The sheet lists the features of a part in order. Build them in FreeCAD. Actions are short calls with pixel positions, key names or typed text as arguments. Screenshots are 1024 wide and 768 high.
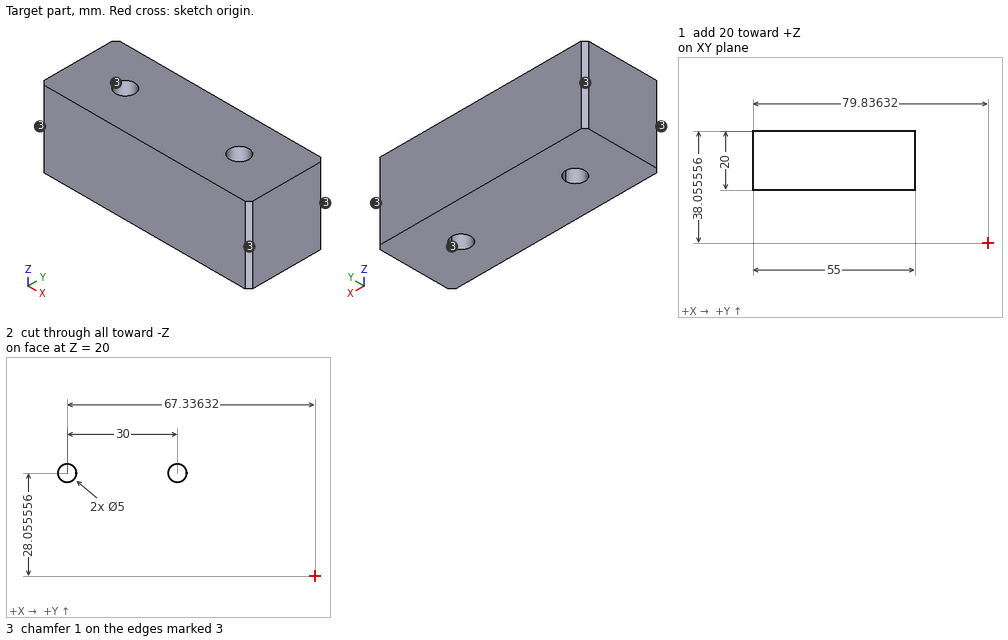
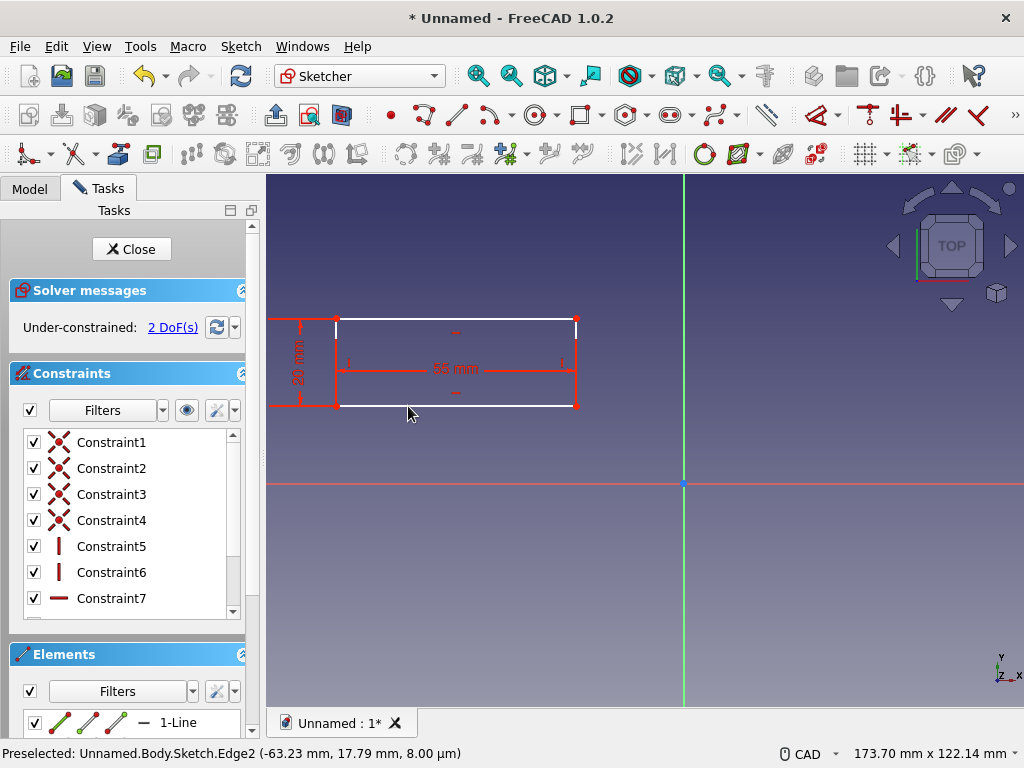
click(336, 319)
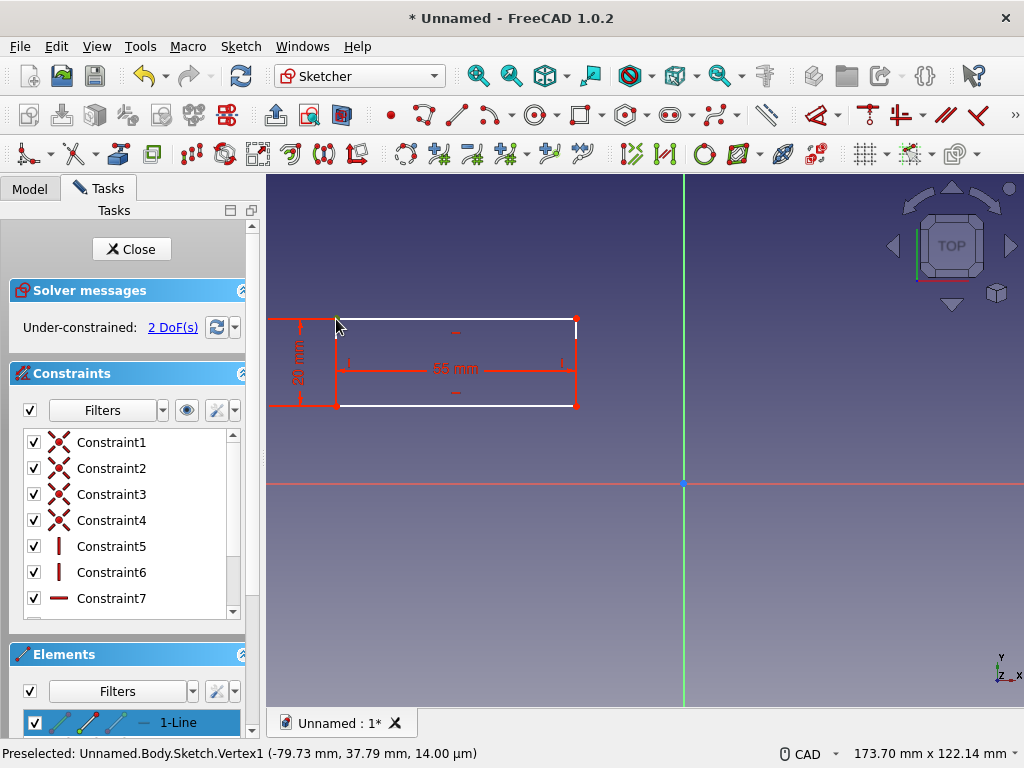
click(838, 116)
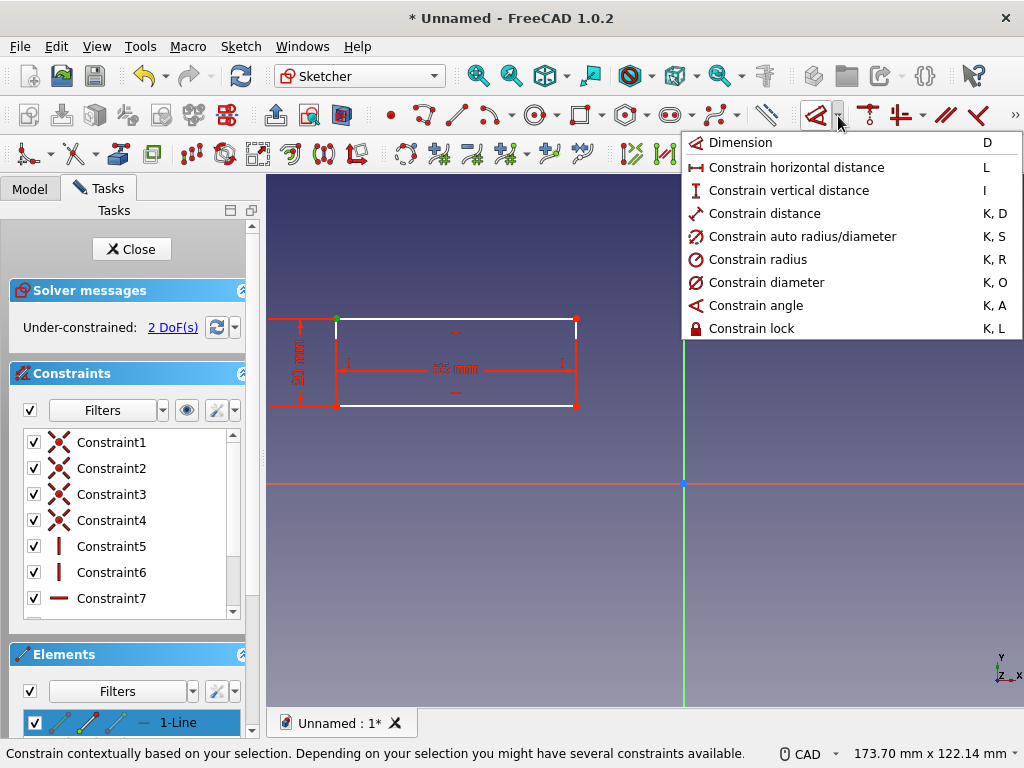
click(852, 168)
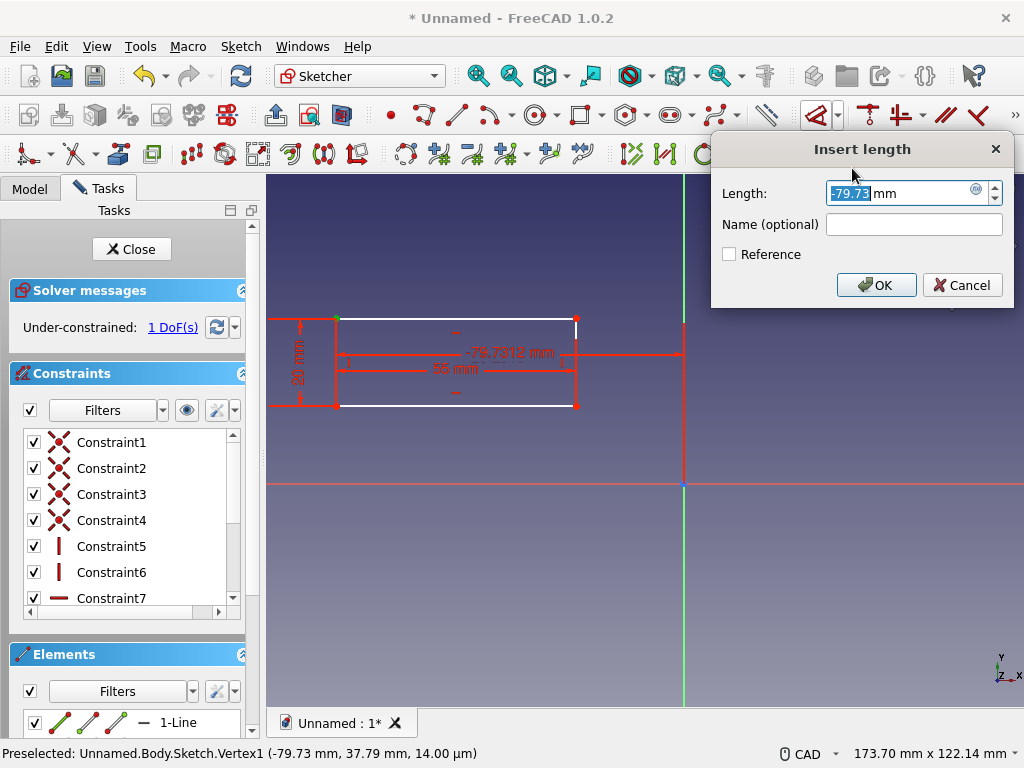
text(-79.83632)
key(Return)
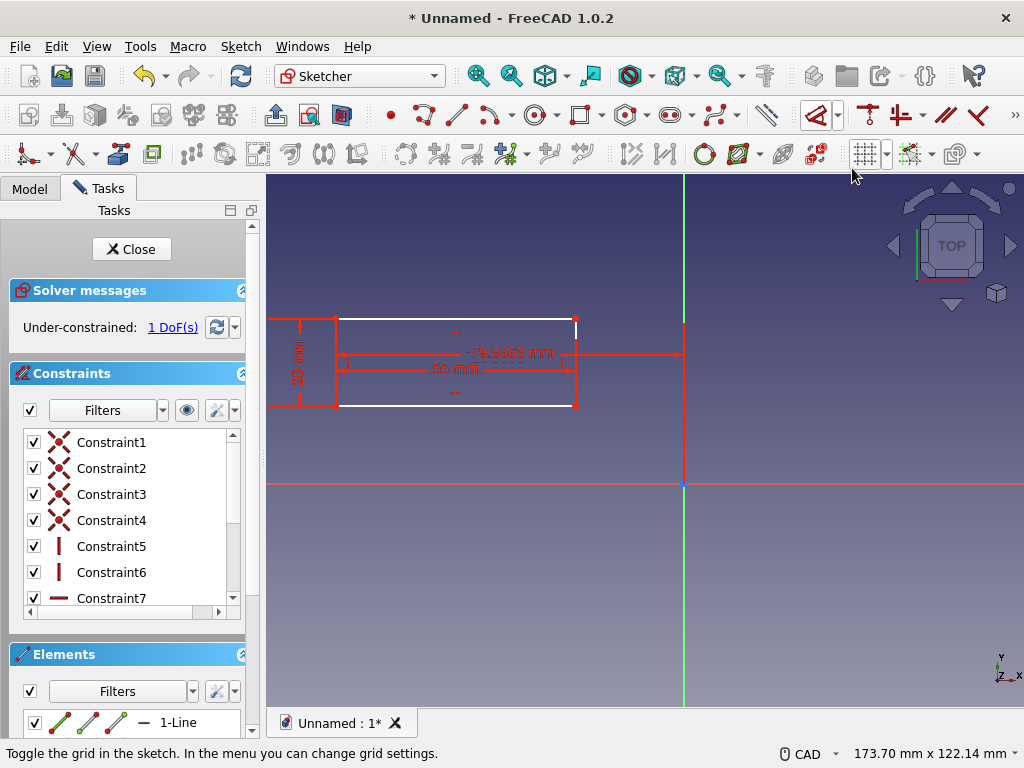
click(336, 319)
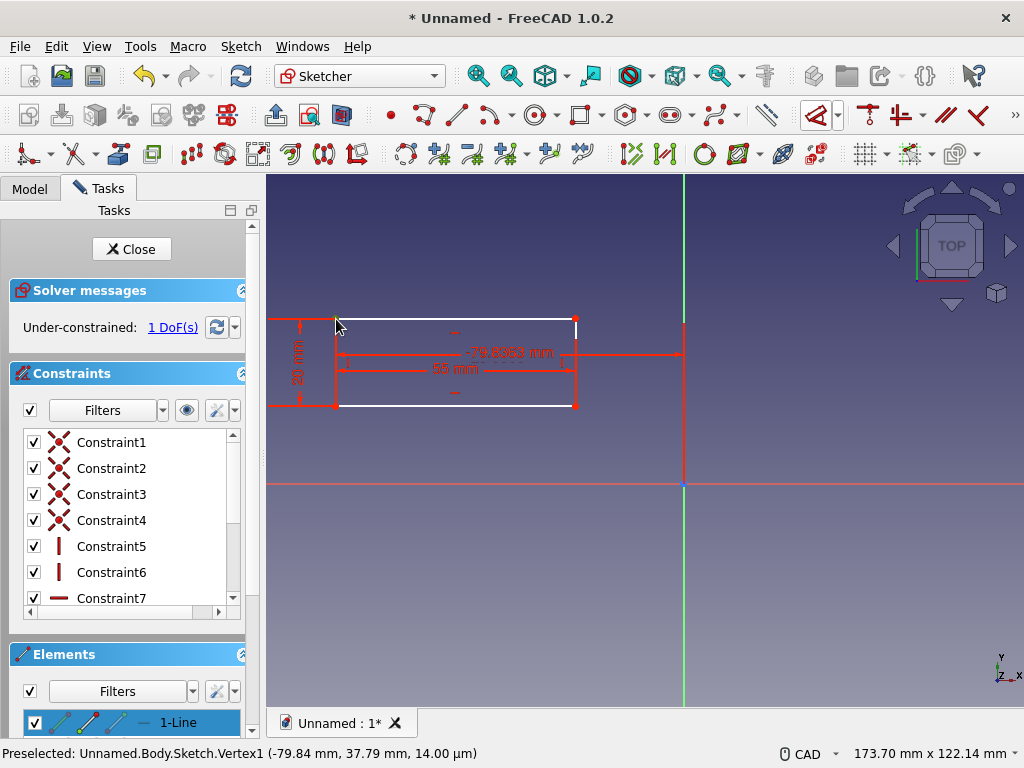
key(i)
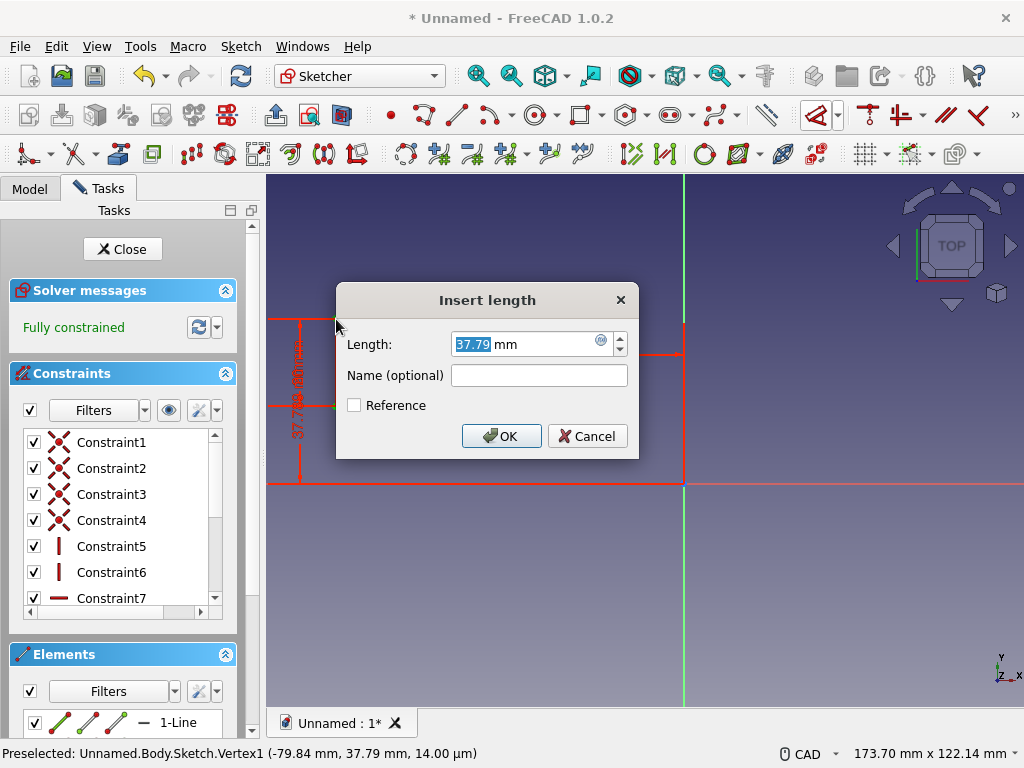
text(38.055556)
key(Return)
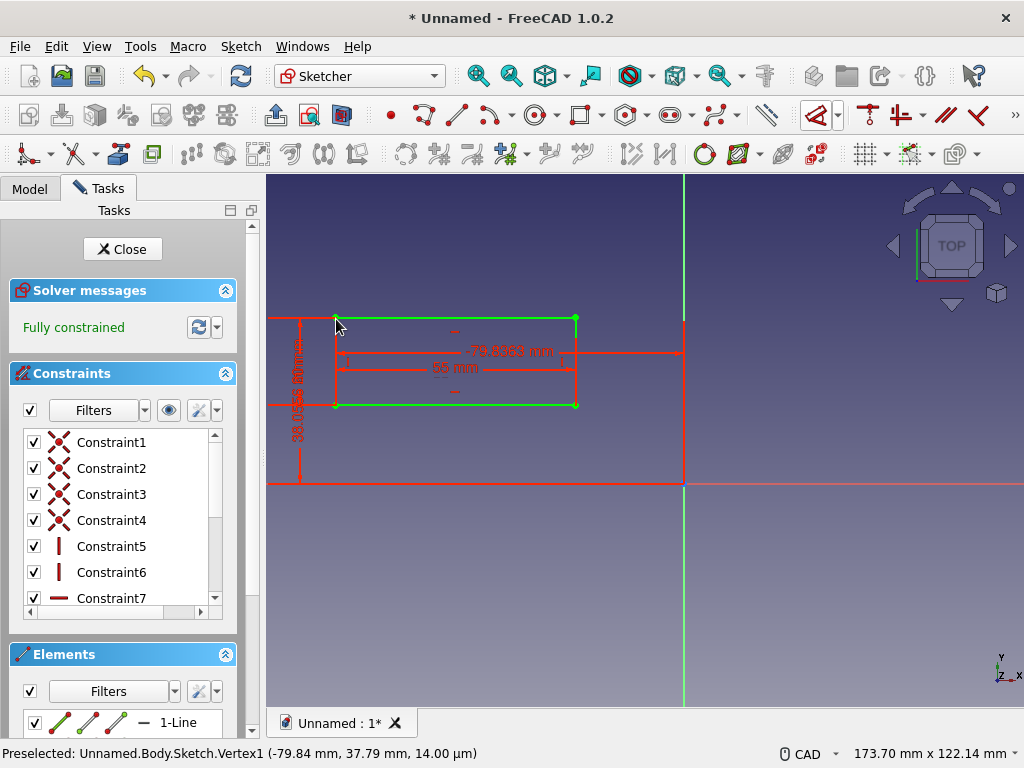
click(123, 249)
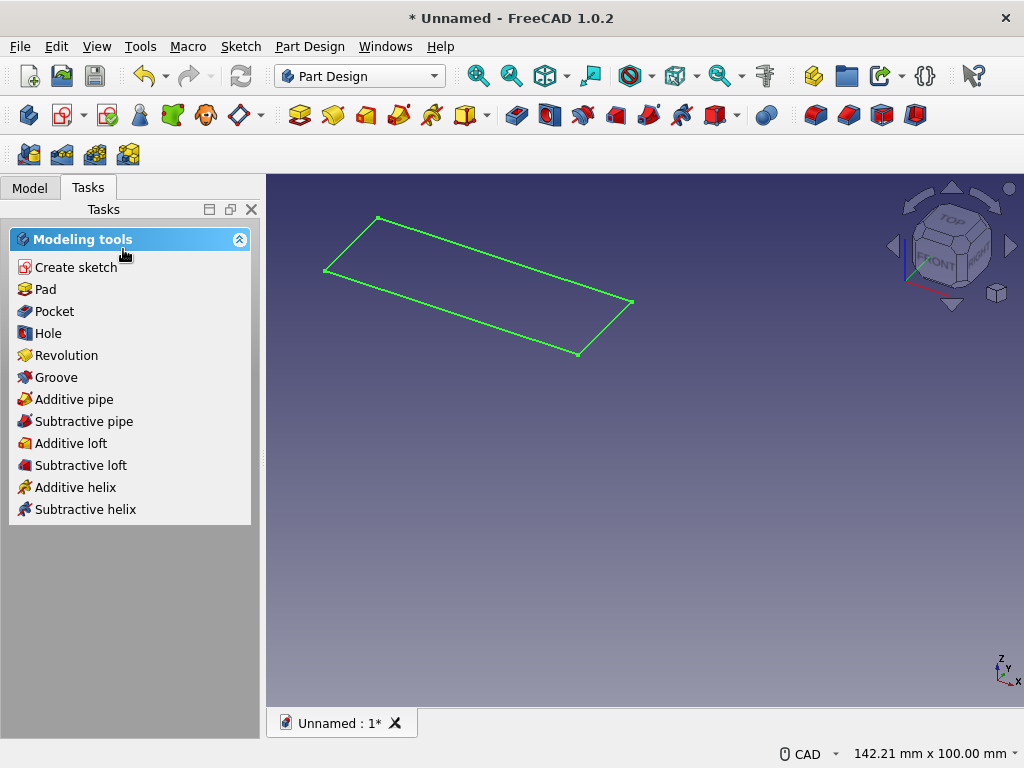
click(300, 116)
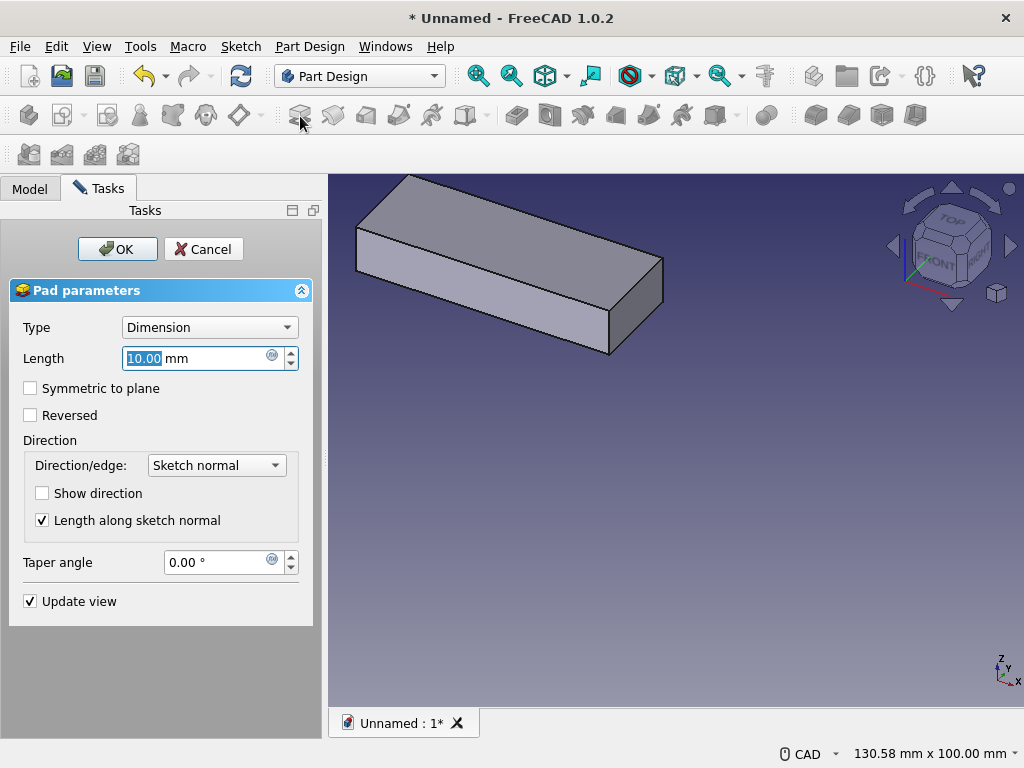
text(20)
key(Tab)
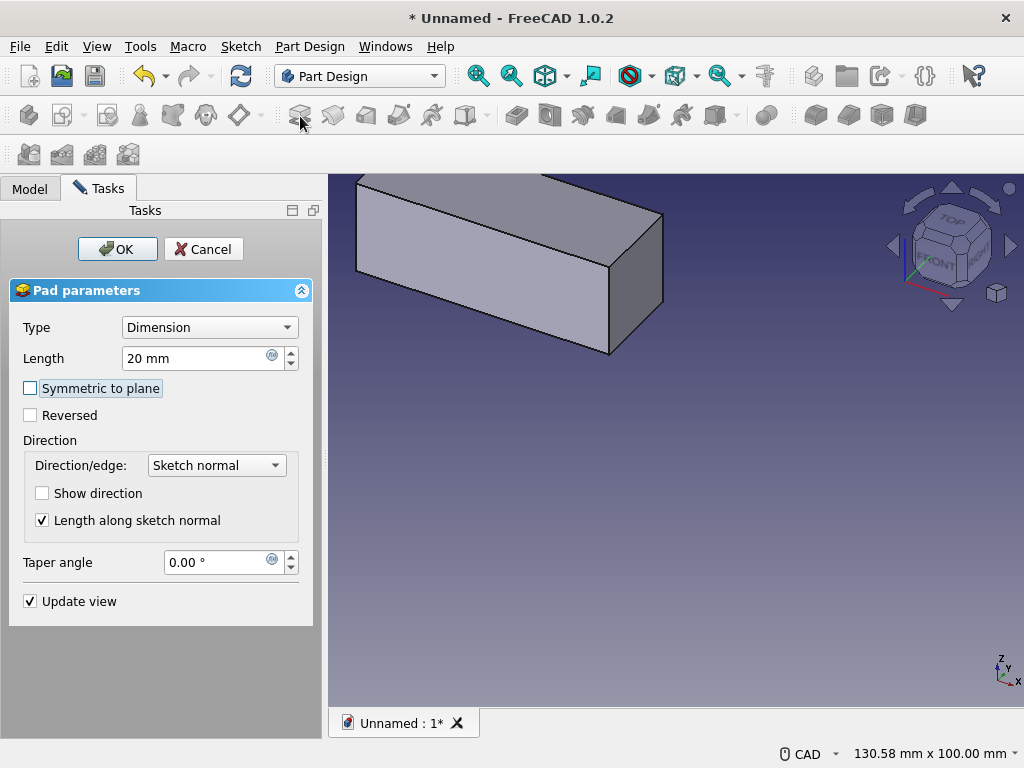
click(118, 249)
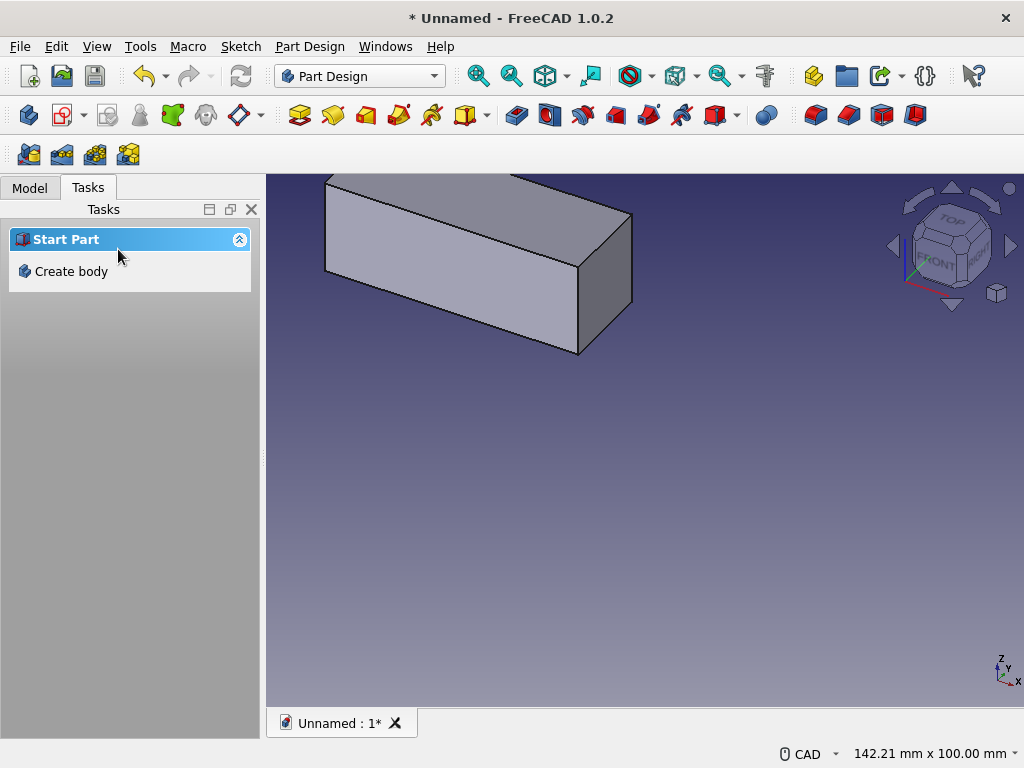
click(479, 76)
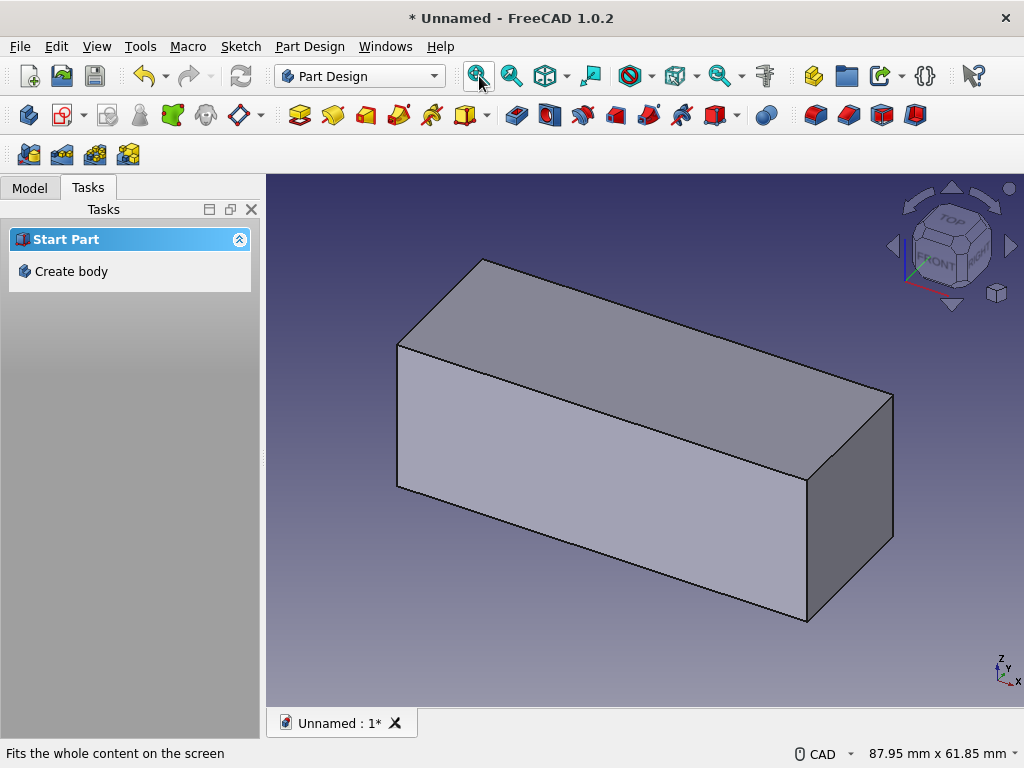
click(762, 408)